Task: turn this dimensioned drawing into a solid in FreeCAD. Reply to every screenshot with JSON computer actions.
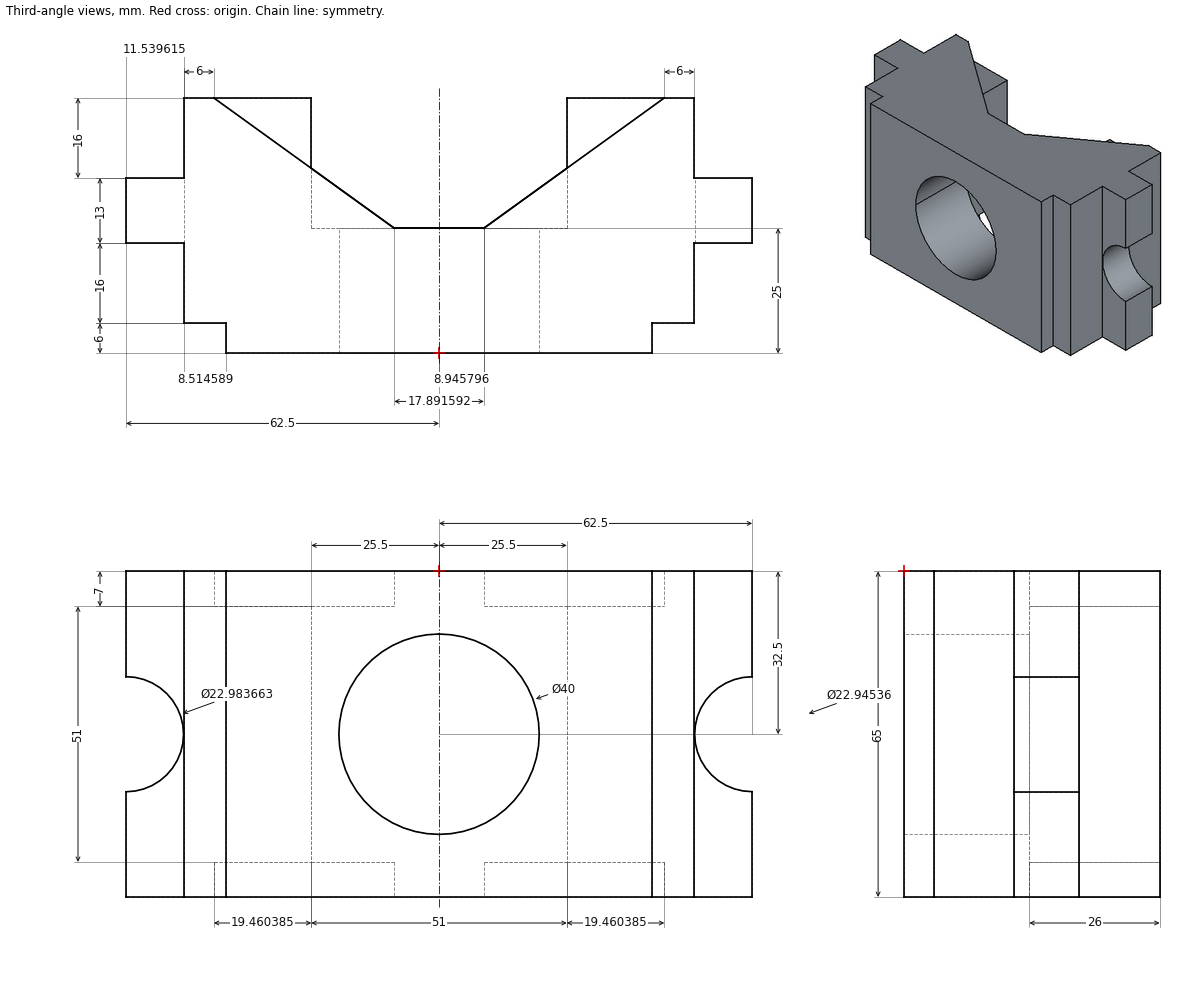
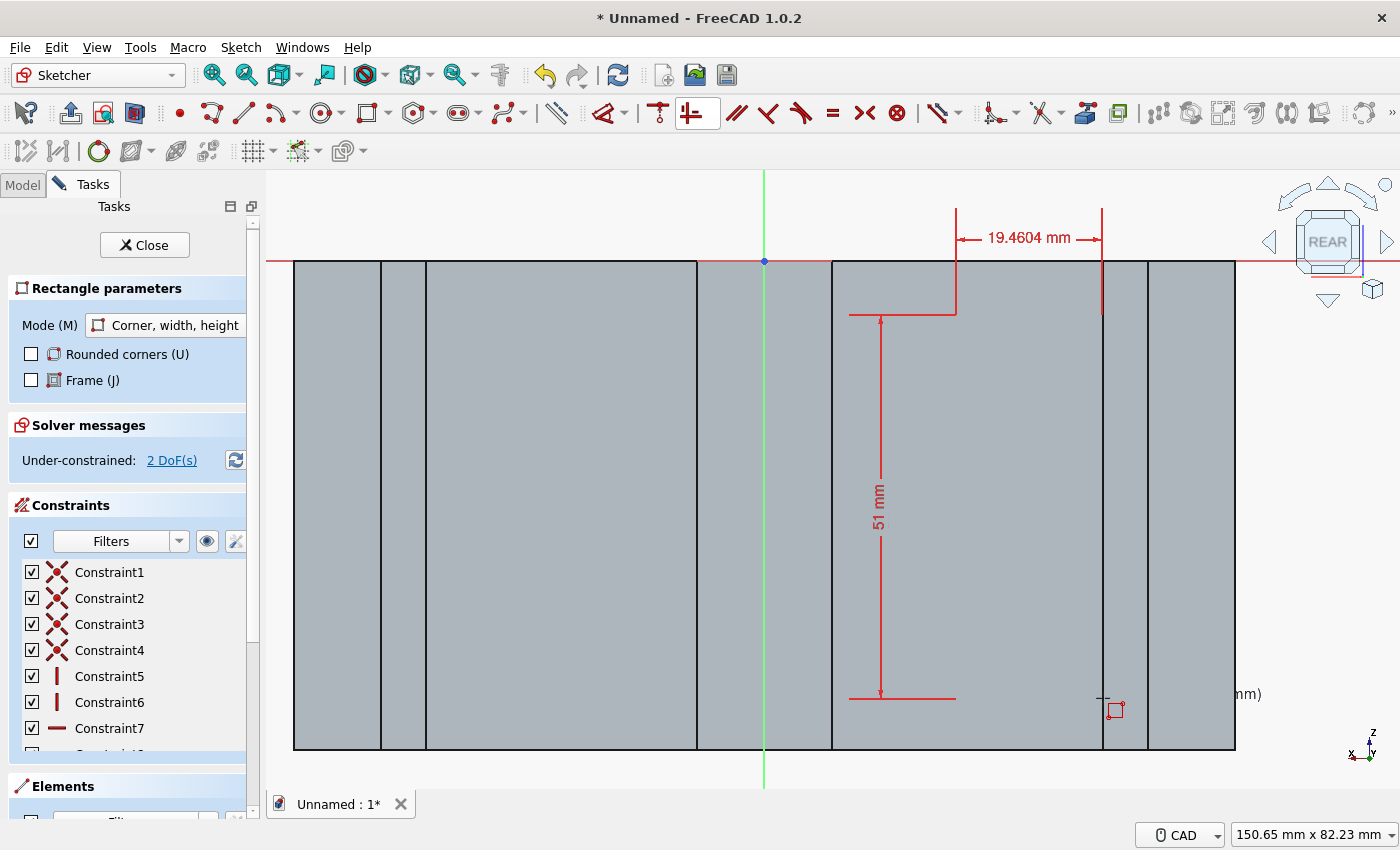
{"action": "left_click", "coordinate": [426, 314]}
{"action": "mouse_move", "coordinate": [572, 698]}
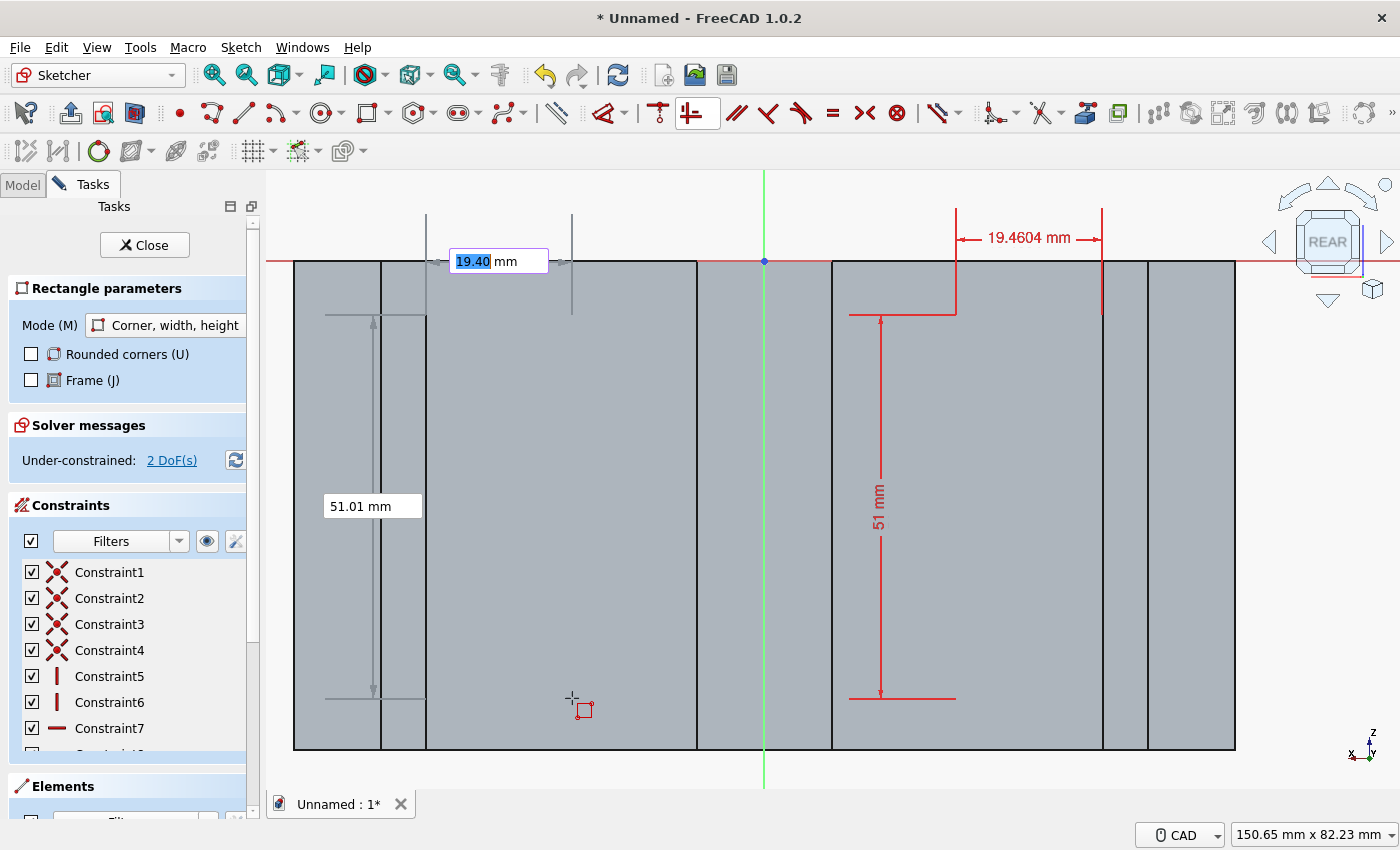
{"action": "type", "text": "19.460385"}
{"action": "key", "text": "Tab"}
{"action": "type", "text": "51"}
{"action": "key", "text": "Return"}
{"action": "key", "text": "Escape"}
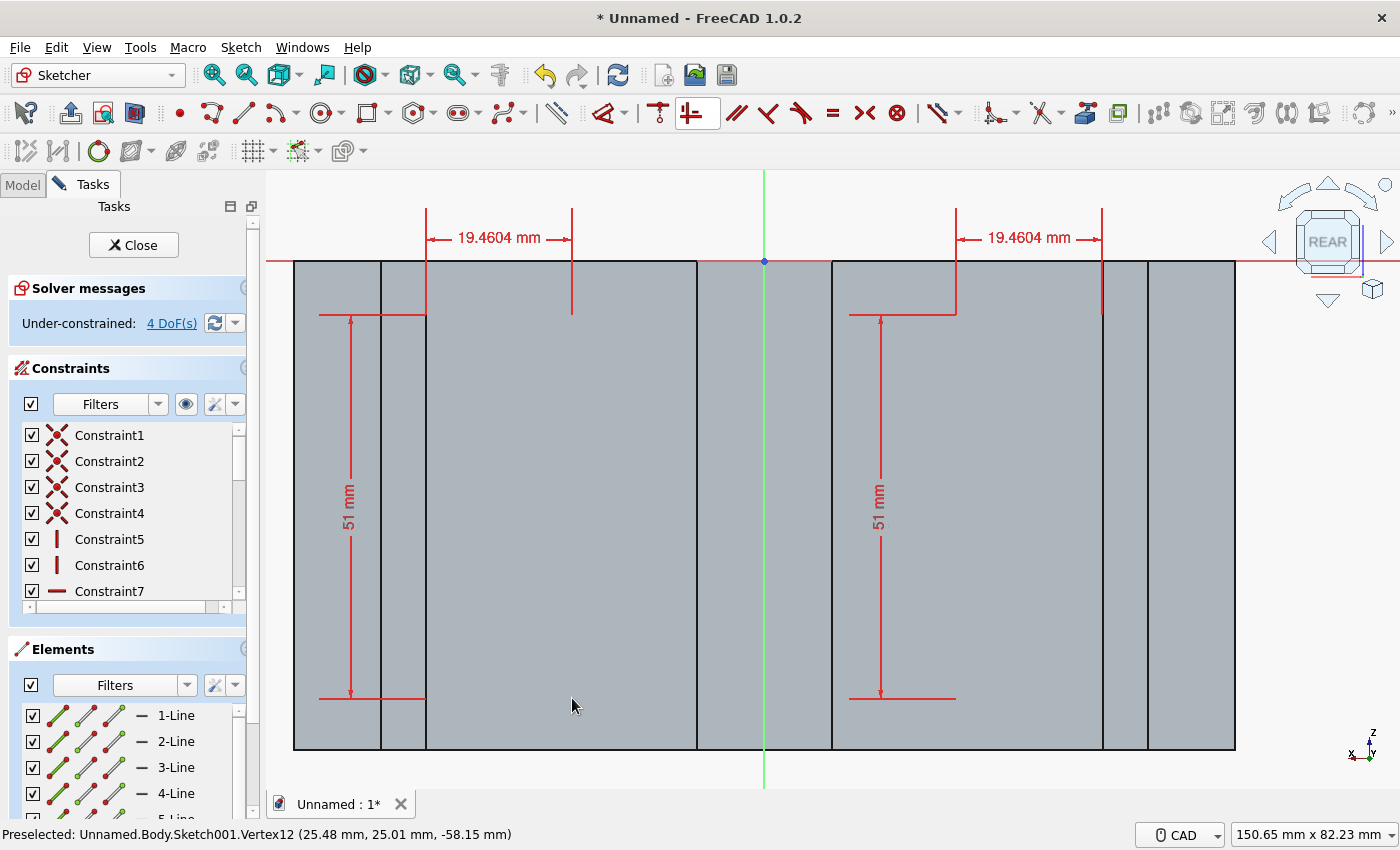
{"action": "left_click", "coordinate": [1102, 315]}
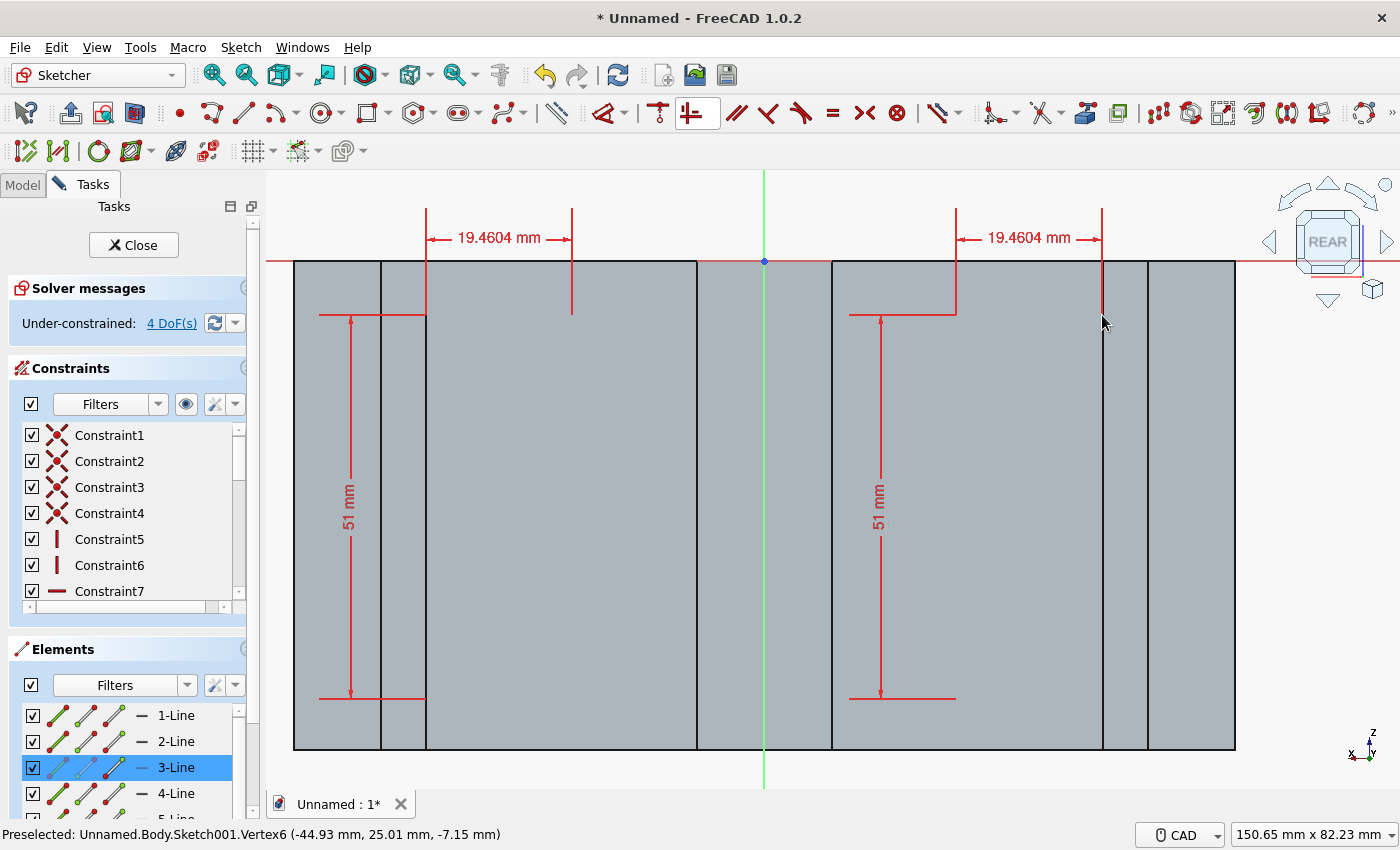
{"action": "left_click", "coordinate": [426, 315]}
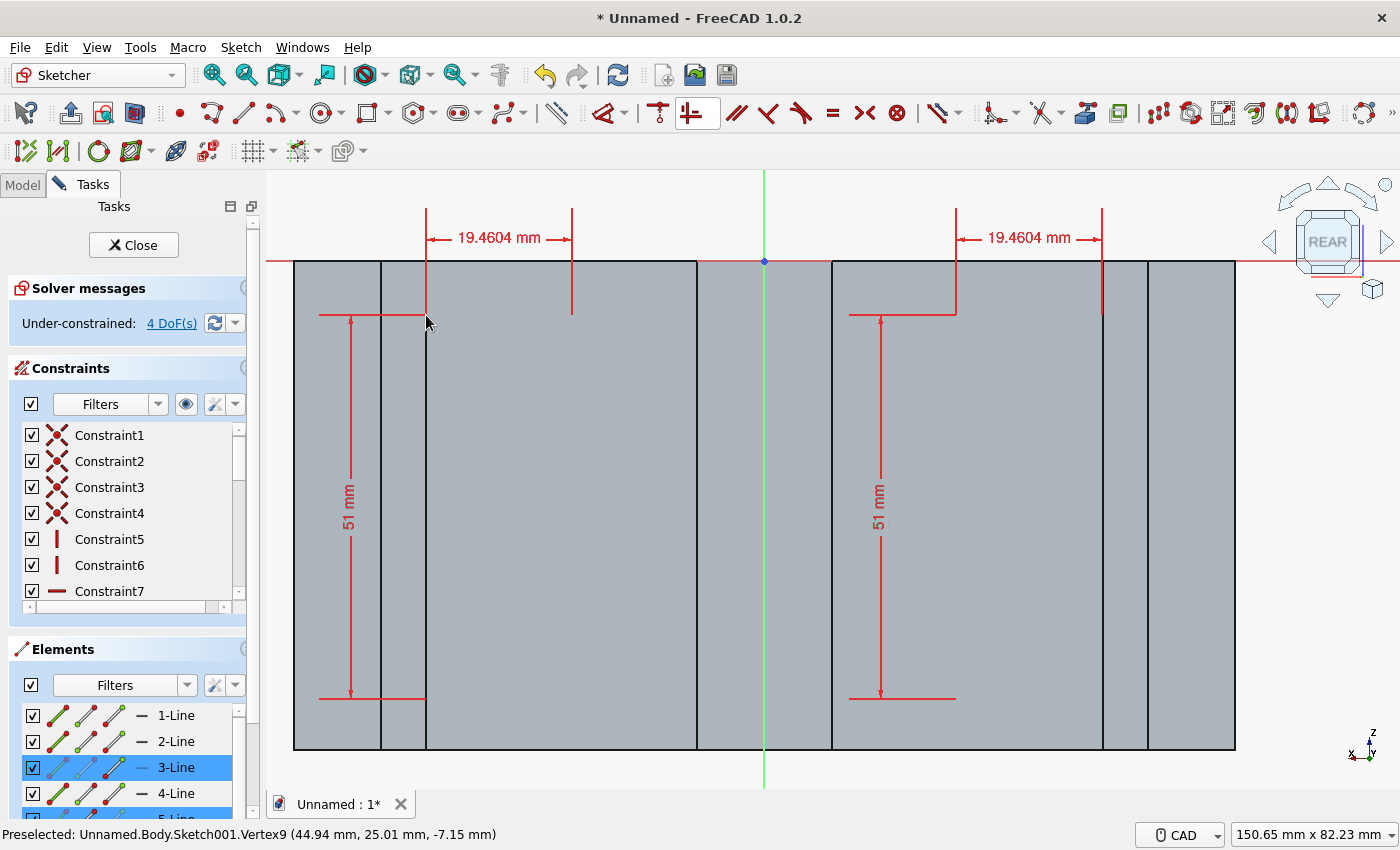
{"action": "left_click", "coordinate": [764, 721]}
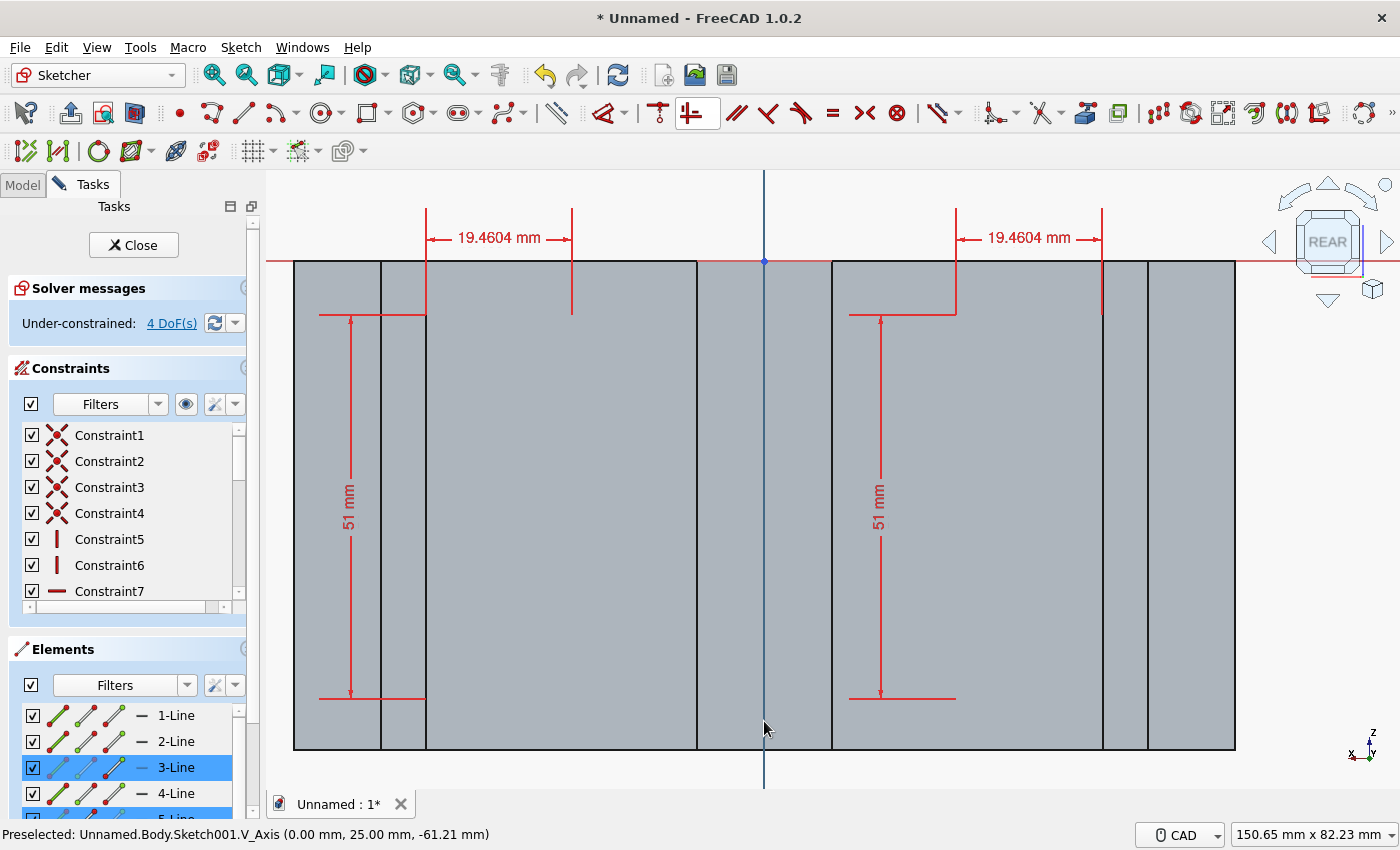
{"action": "left_click", "coordinate": [866, 114]}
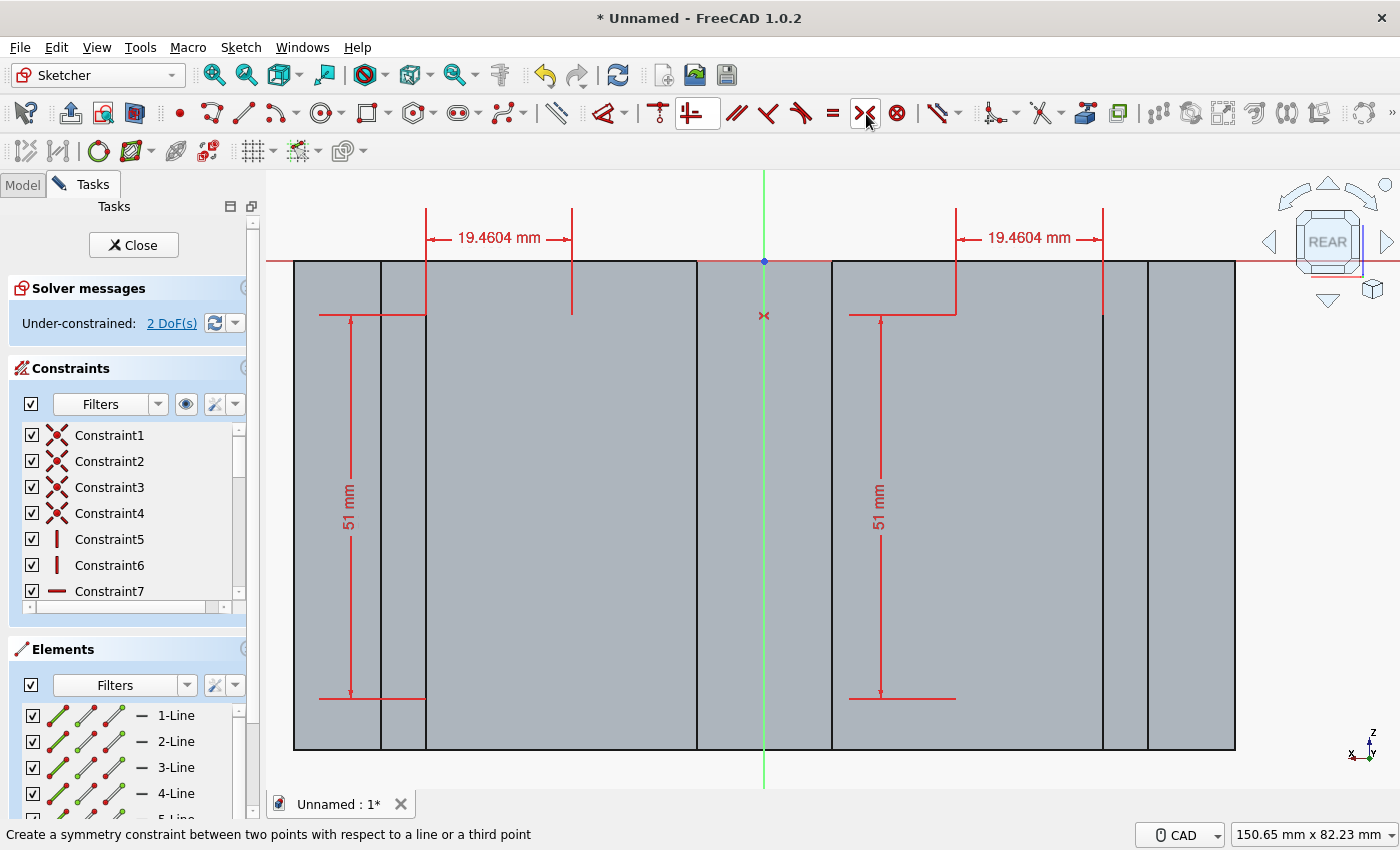
{"action": "left_click", "coordinate": [604, 114]}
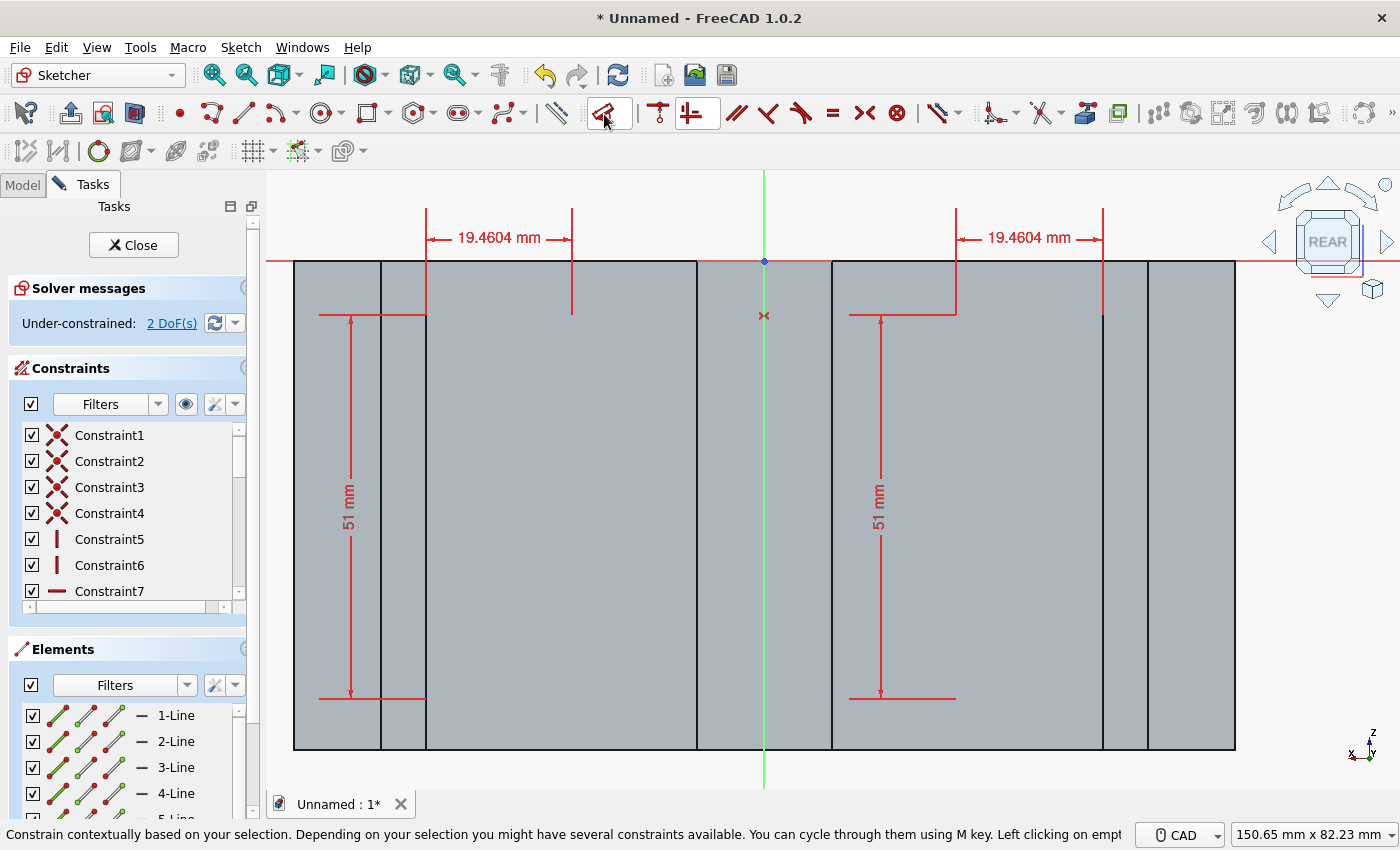
{"action": "left_click", "coordinate": [956, 315]}
{"action": "left_click", "coordinate": [990, 288]}